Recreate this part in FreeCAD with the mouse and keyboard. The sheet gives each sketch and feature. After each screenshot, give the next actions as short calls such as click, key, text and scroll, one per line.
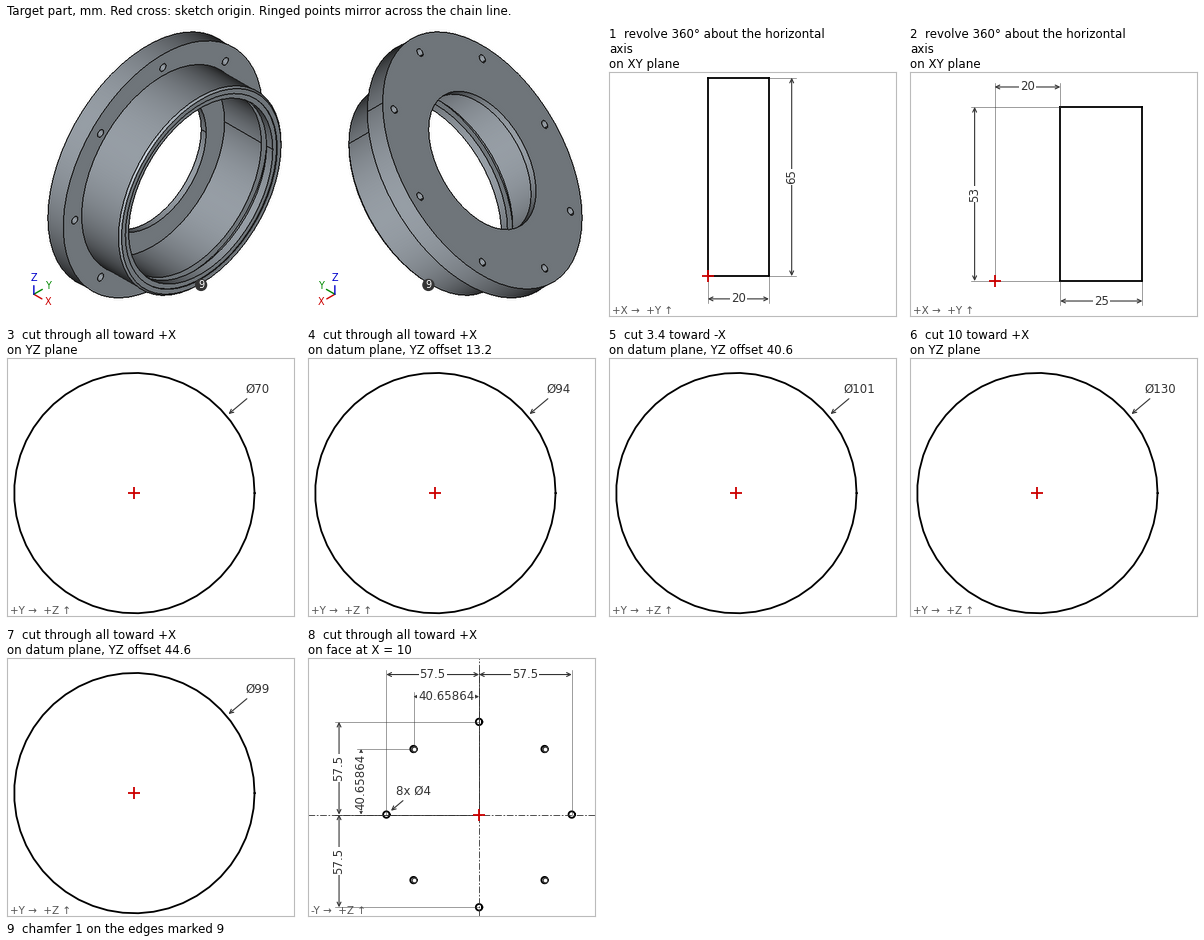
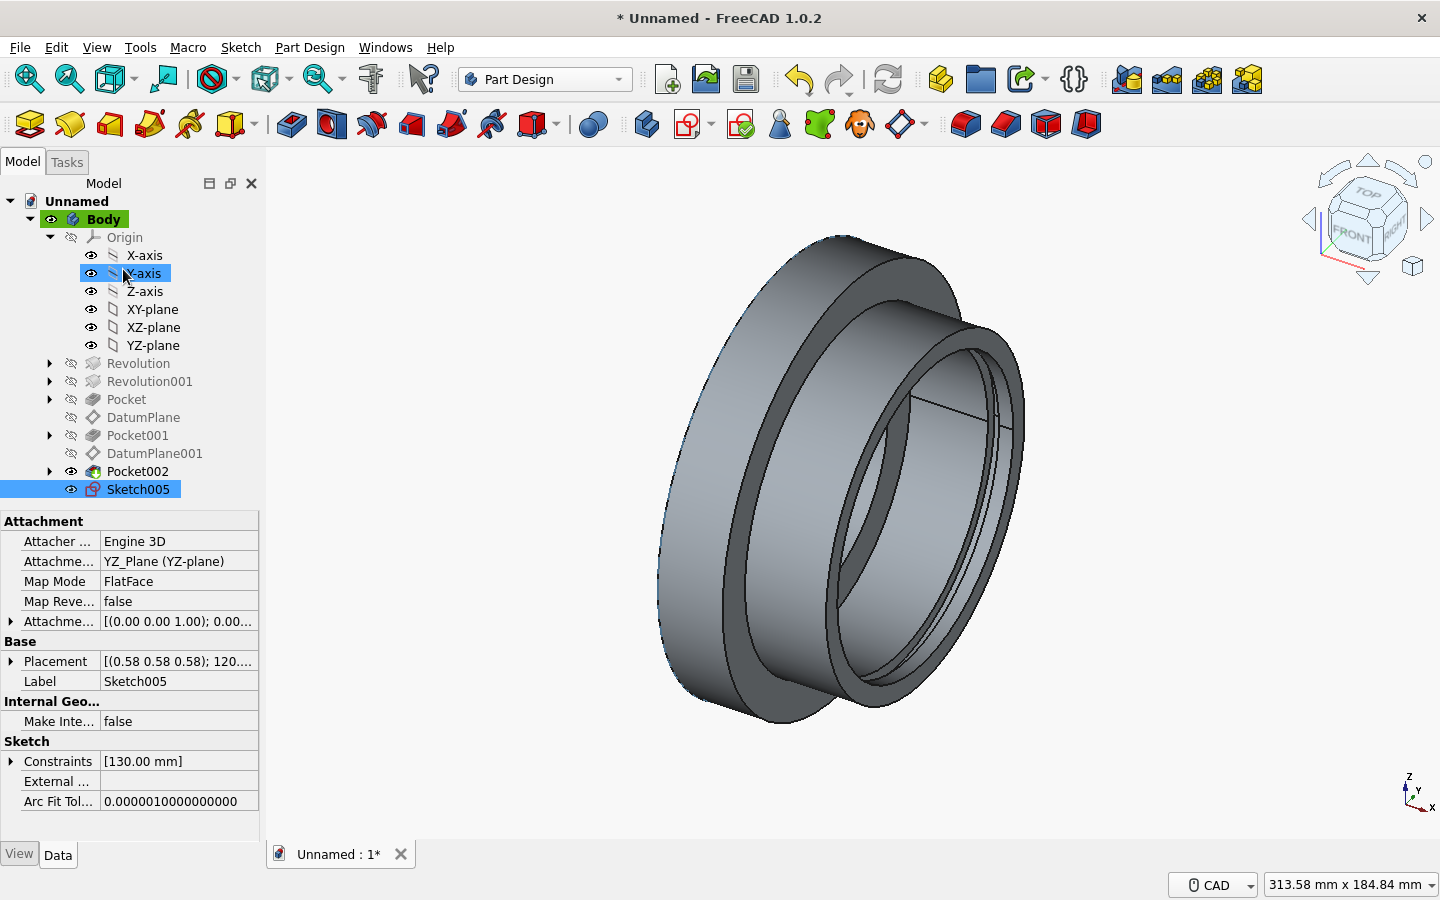
click(292, 124)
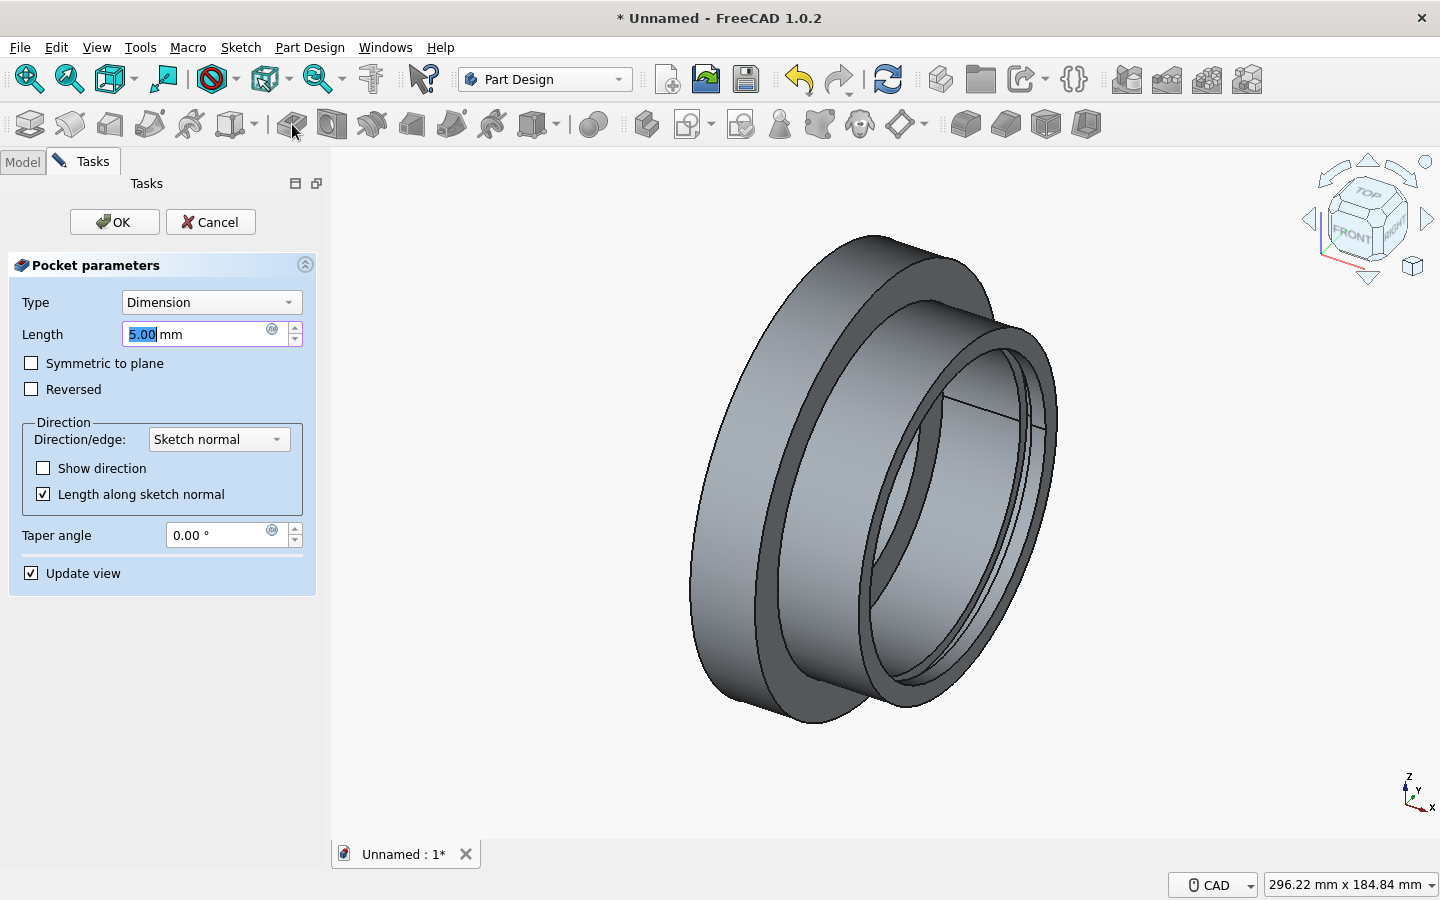
text(10)
key(Tab)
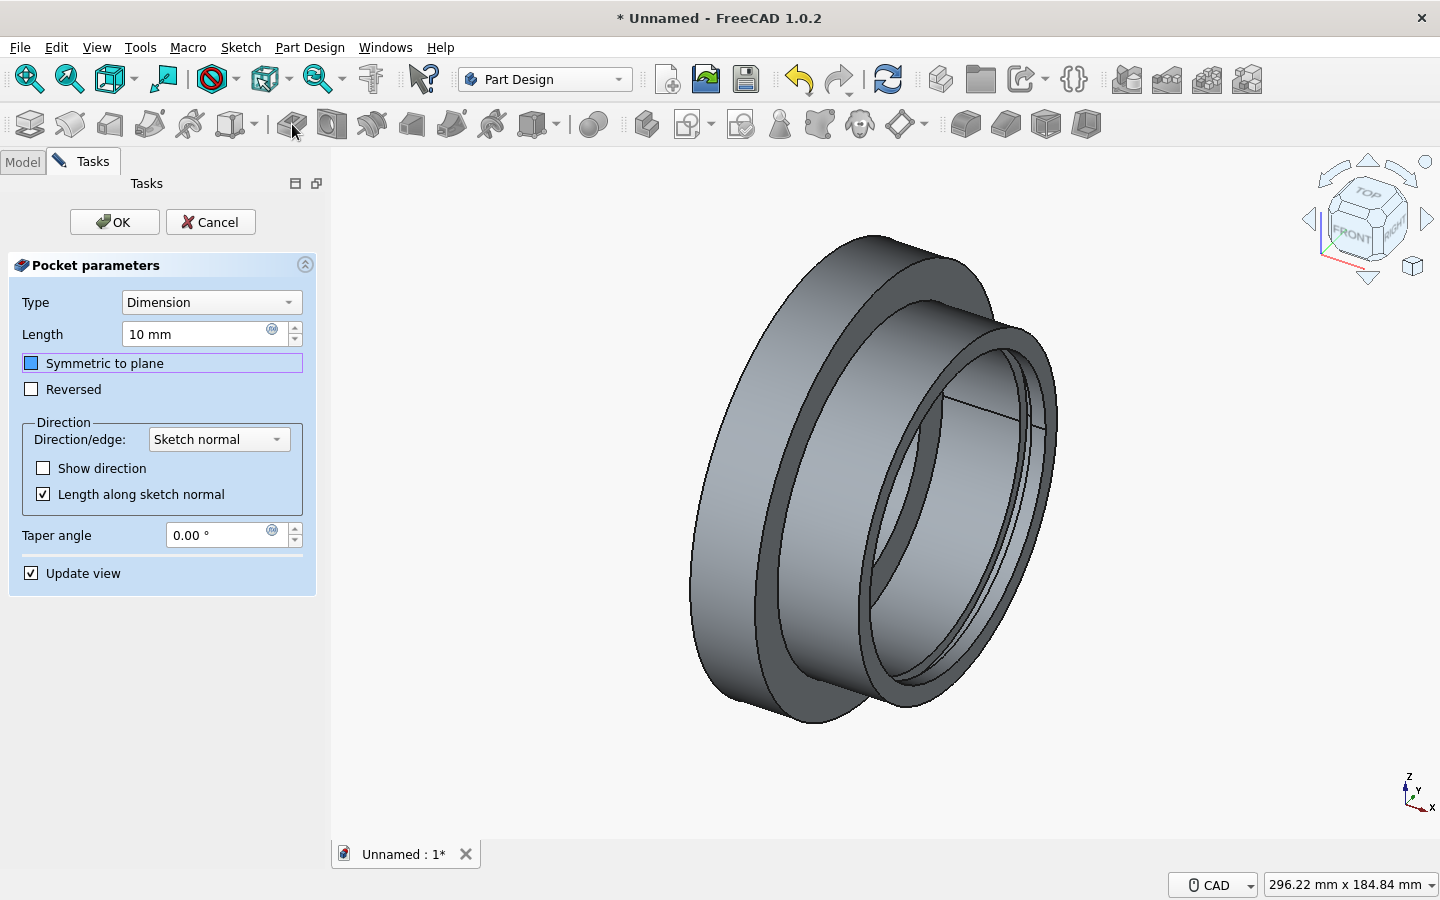
click(30, 389)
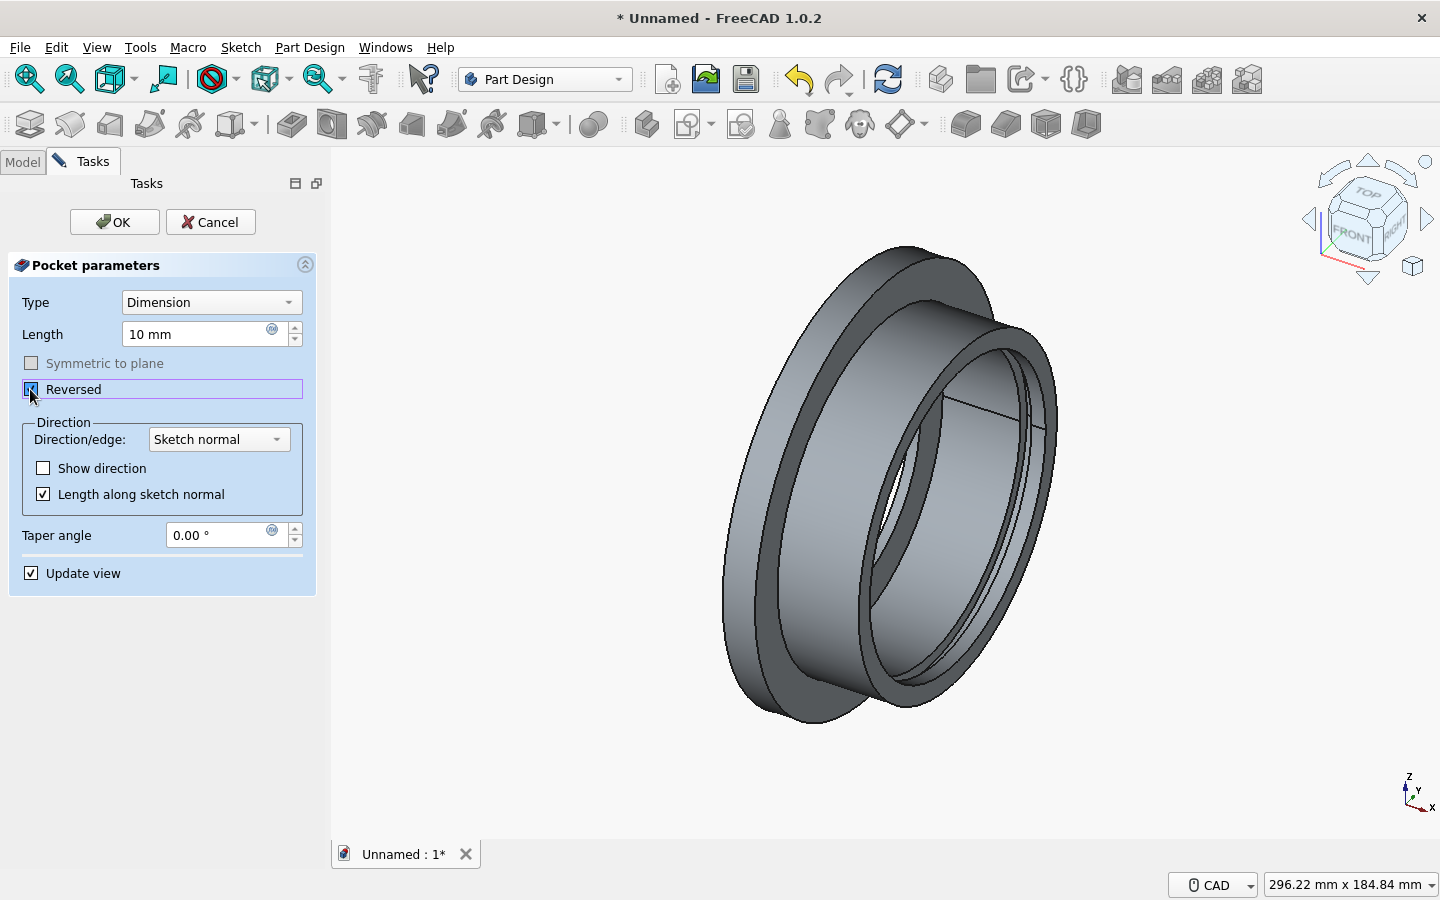
click(115, 222)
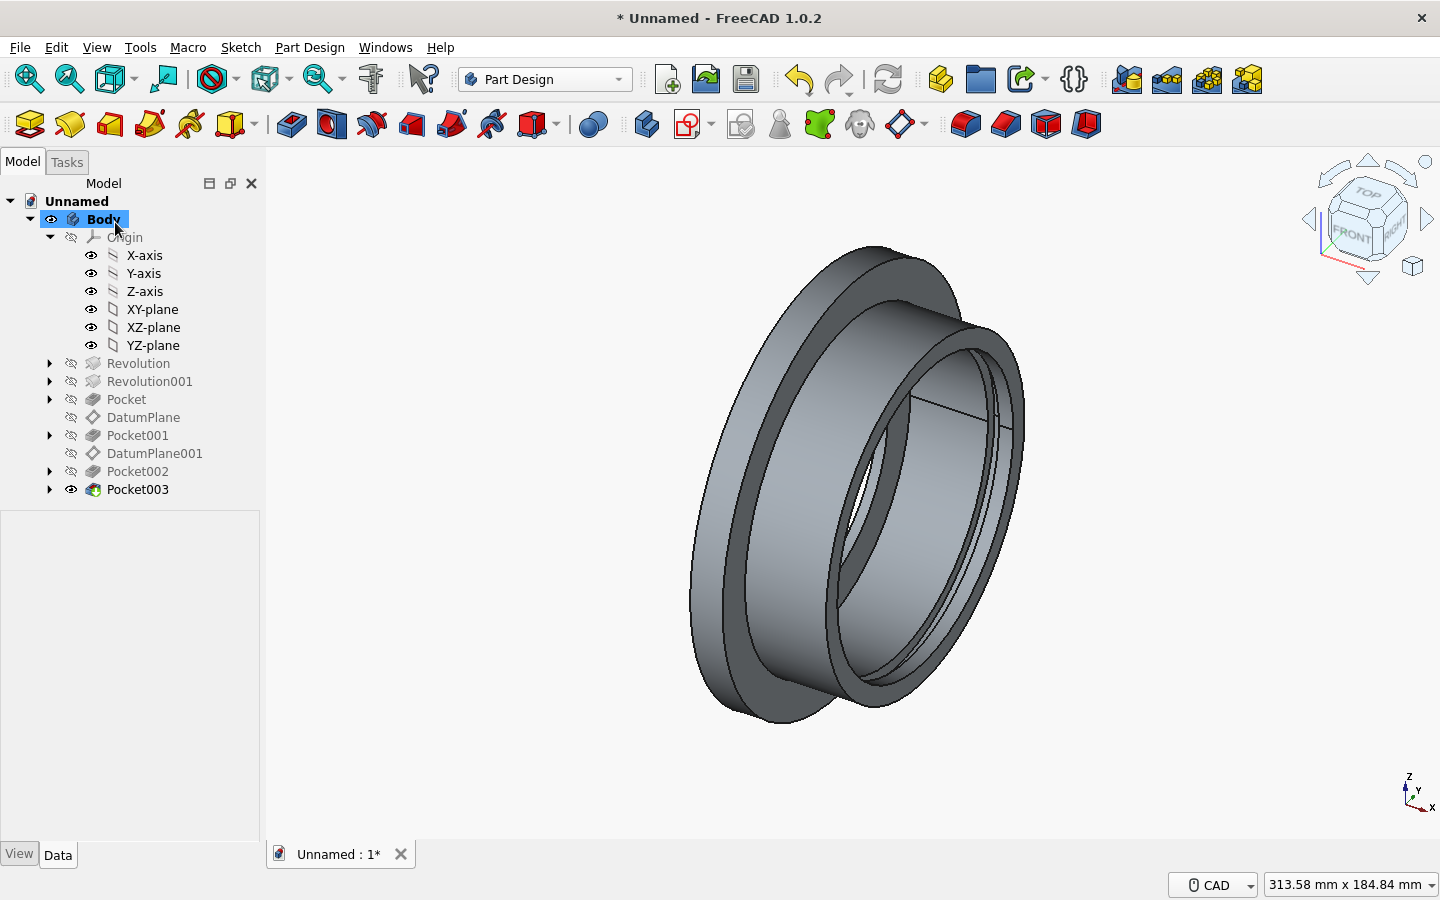
click(136, 345)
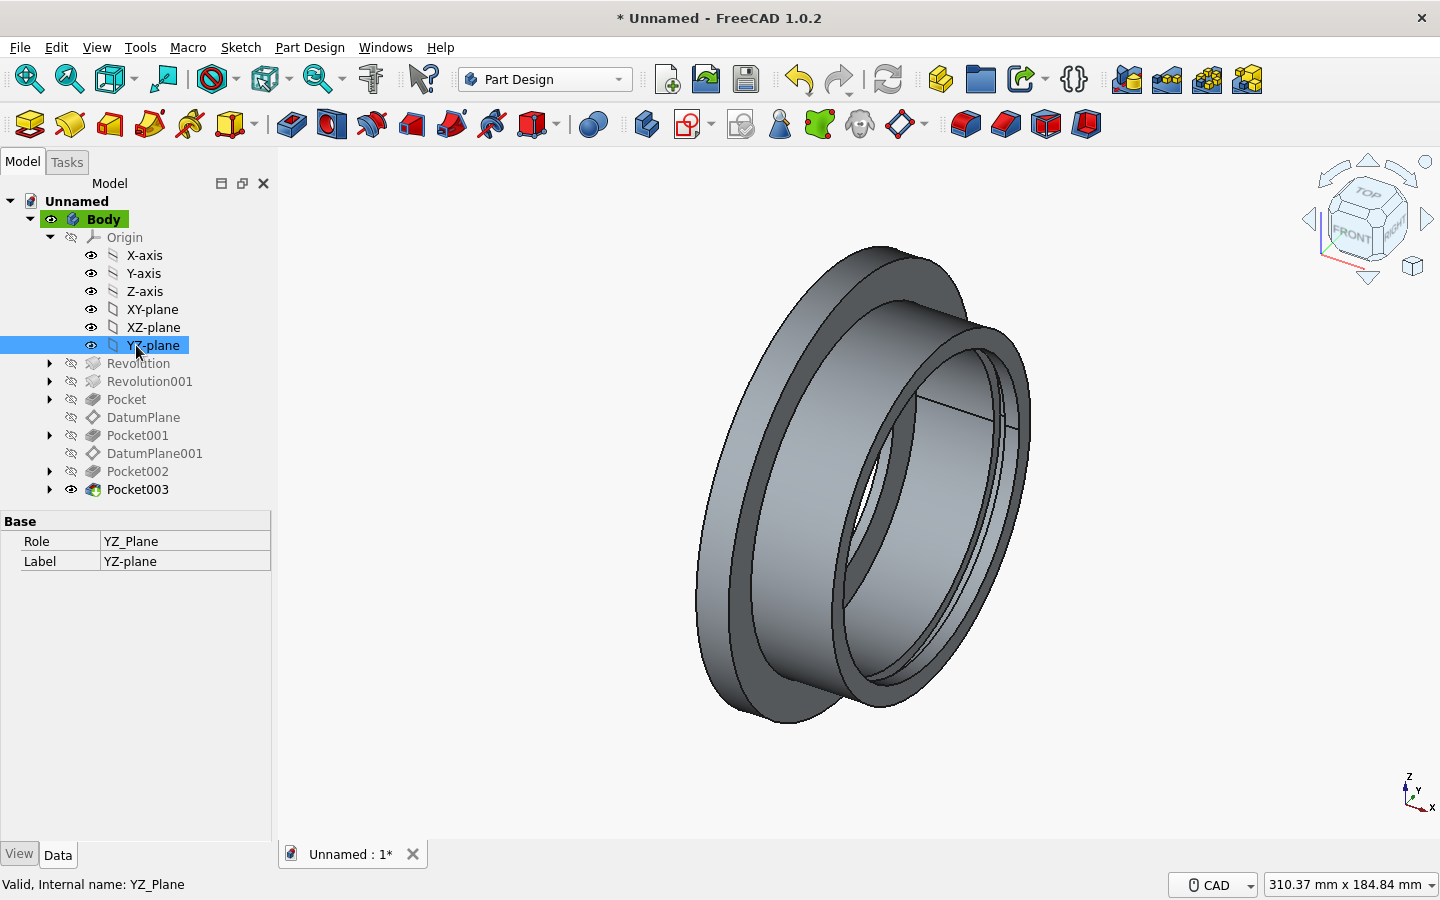
click(900, 124)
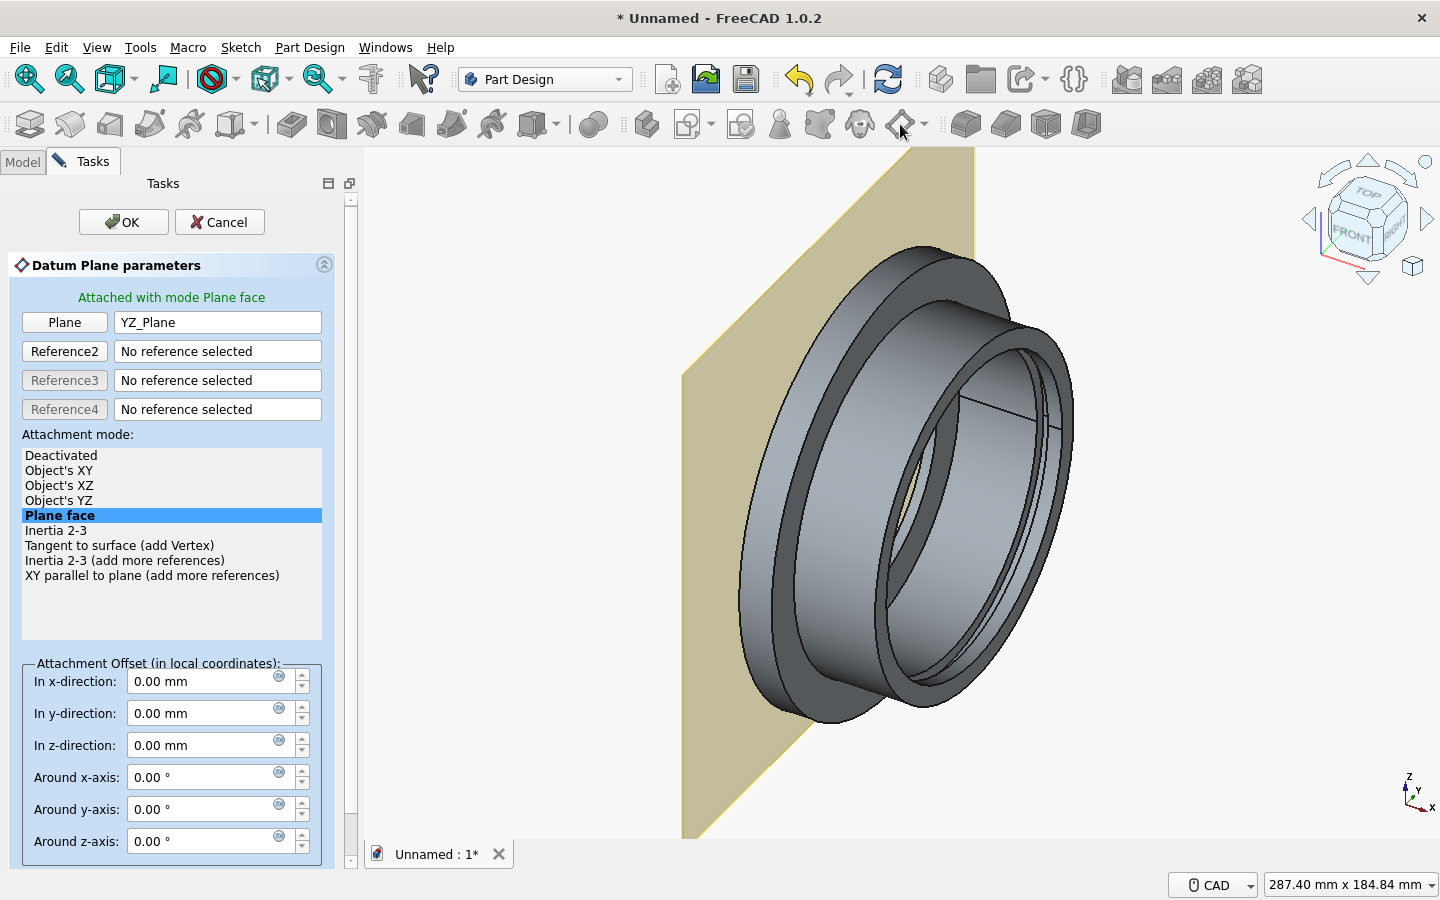
triple_click(210, 745)